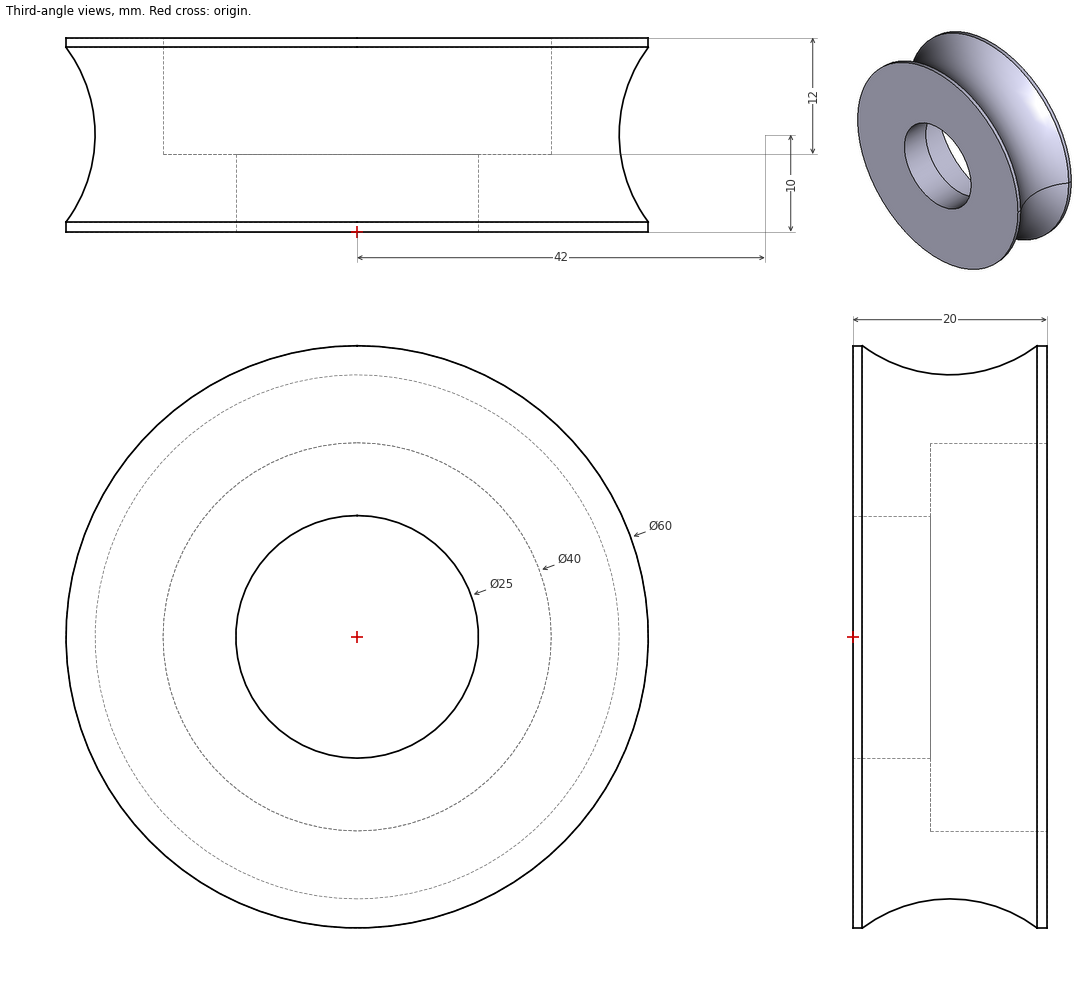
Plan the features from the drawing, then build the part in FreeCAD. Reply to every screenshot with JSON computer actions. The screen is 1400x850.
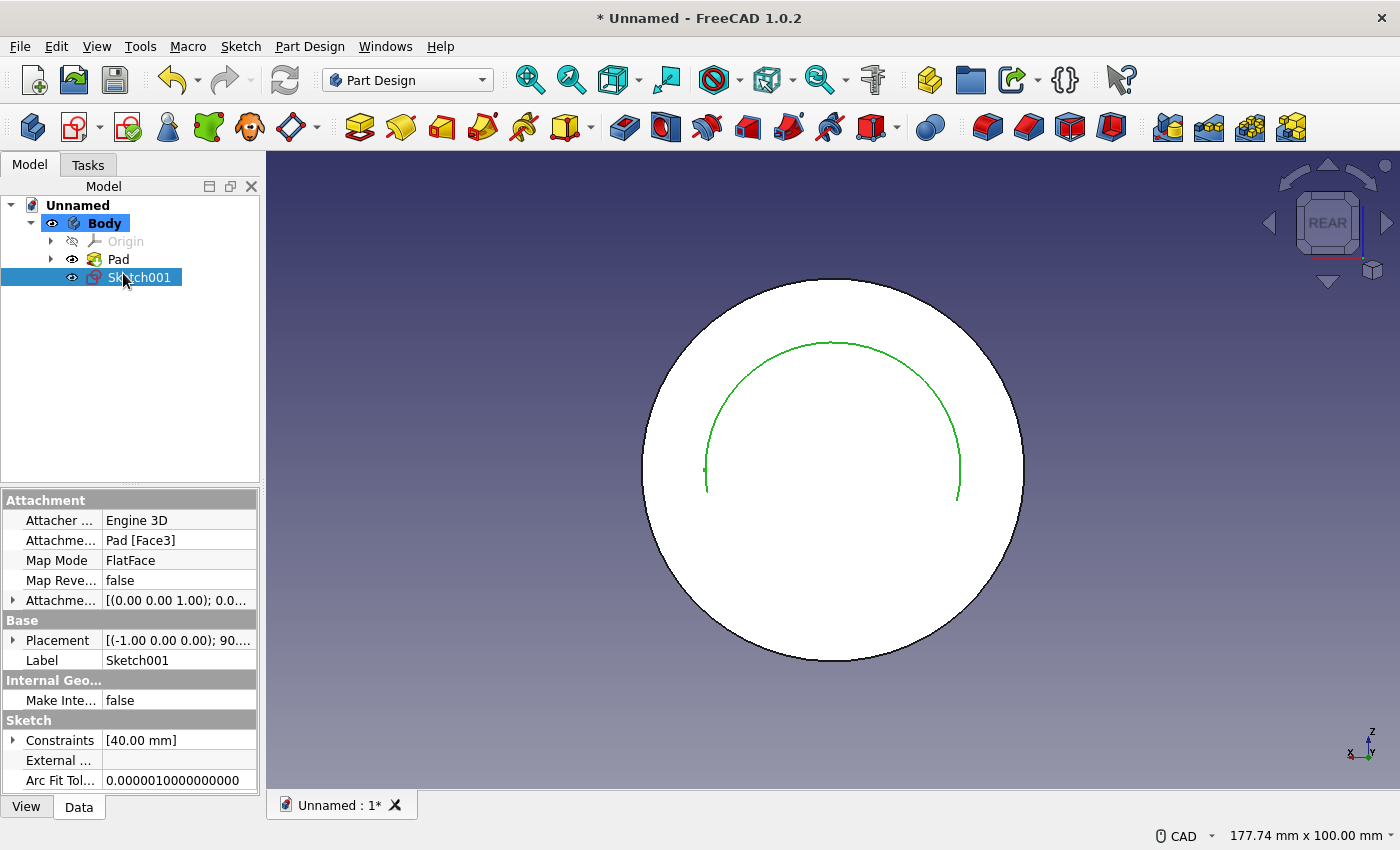
{"action": "left_click", "coordinate": [625, 128]}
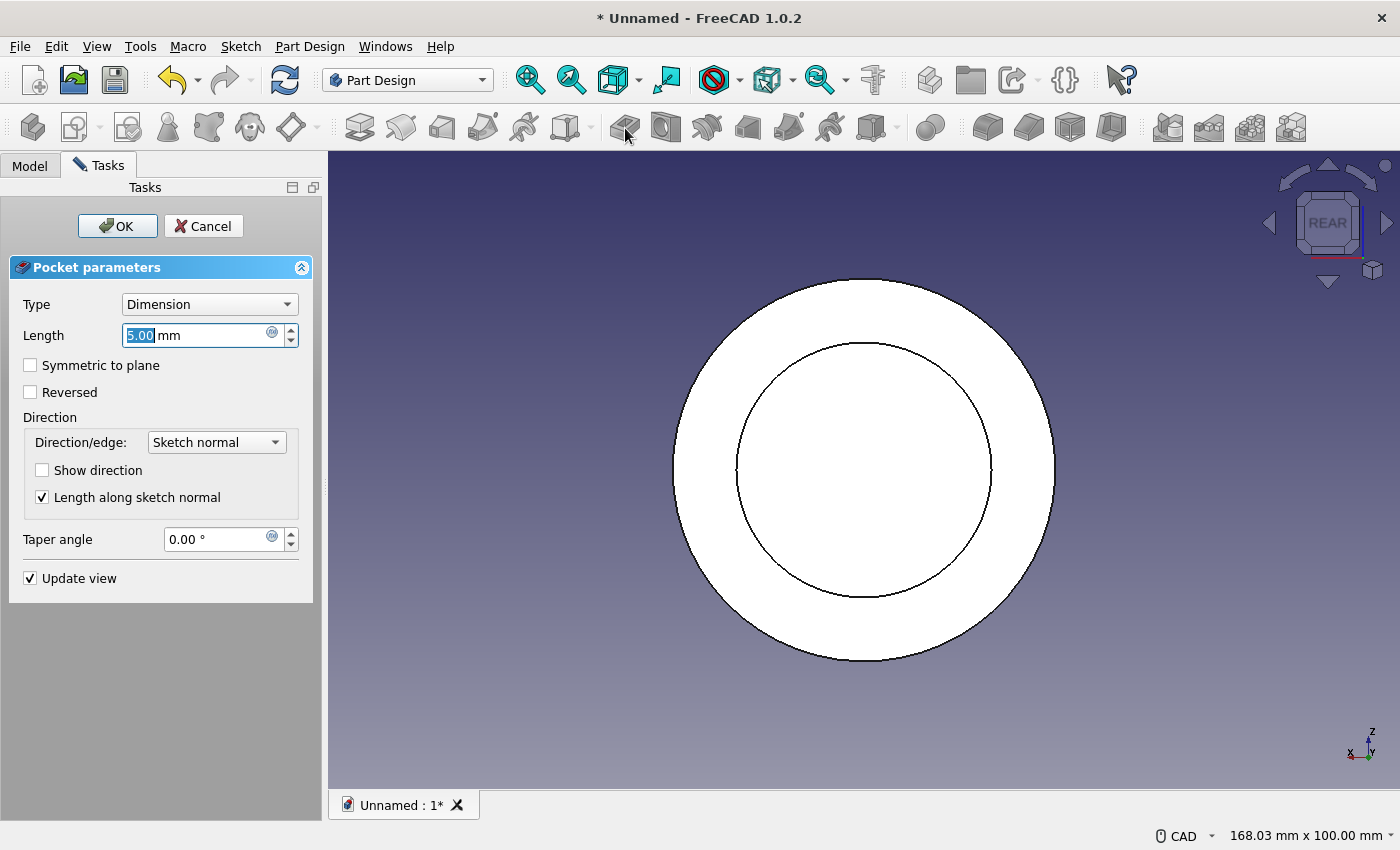
{"action": "type", "text": "12"}
{"action": "key", "text": "Tab"}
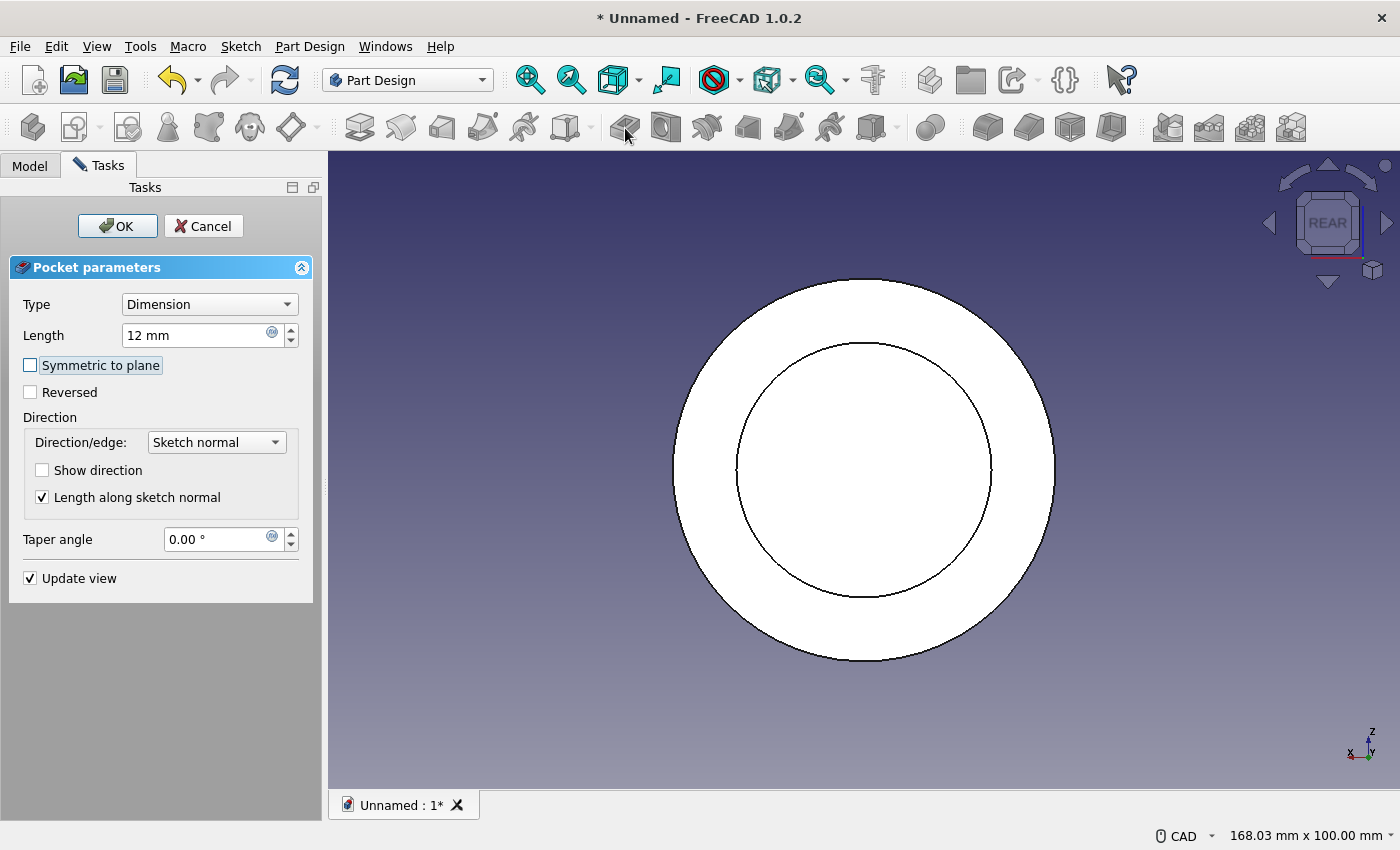
{"action": "left_click", "coordinate": [118, 226]}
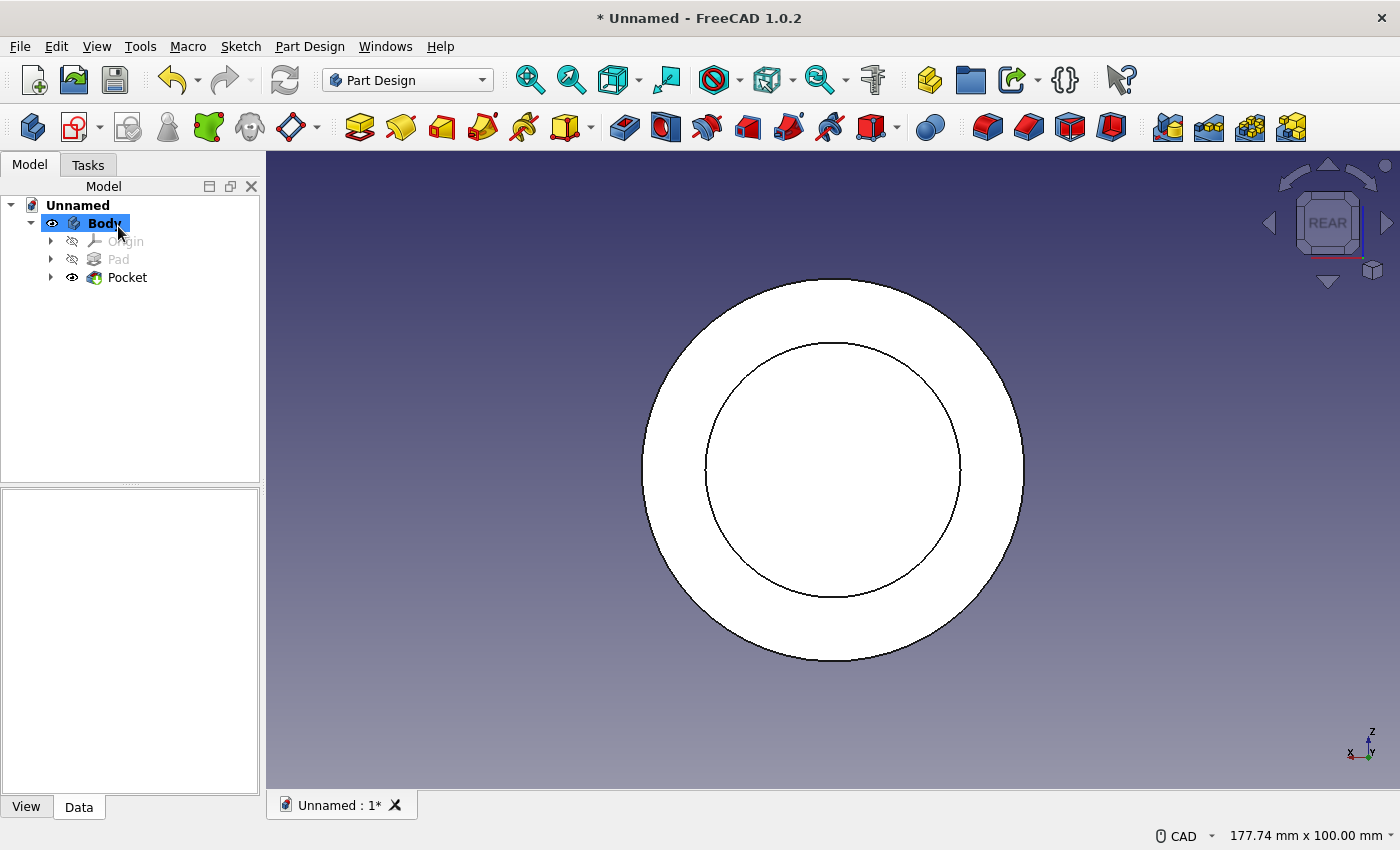
{"action": "left_click", "coordinate": [833, 469]}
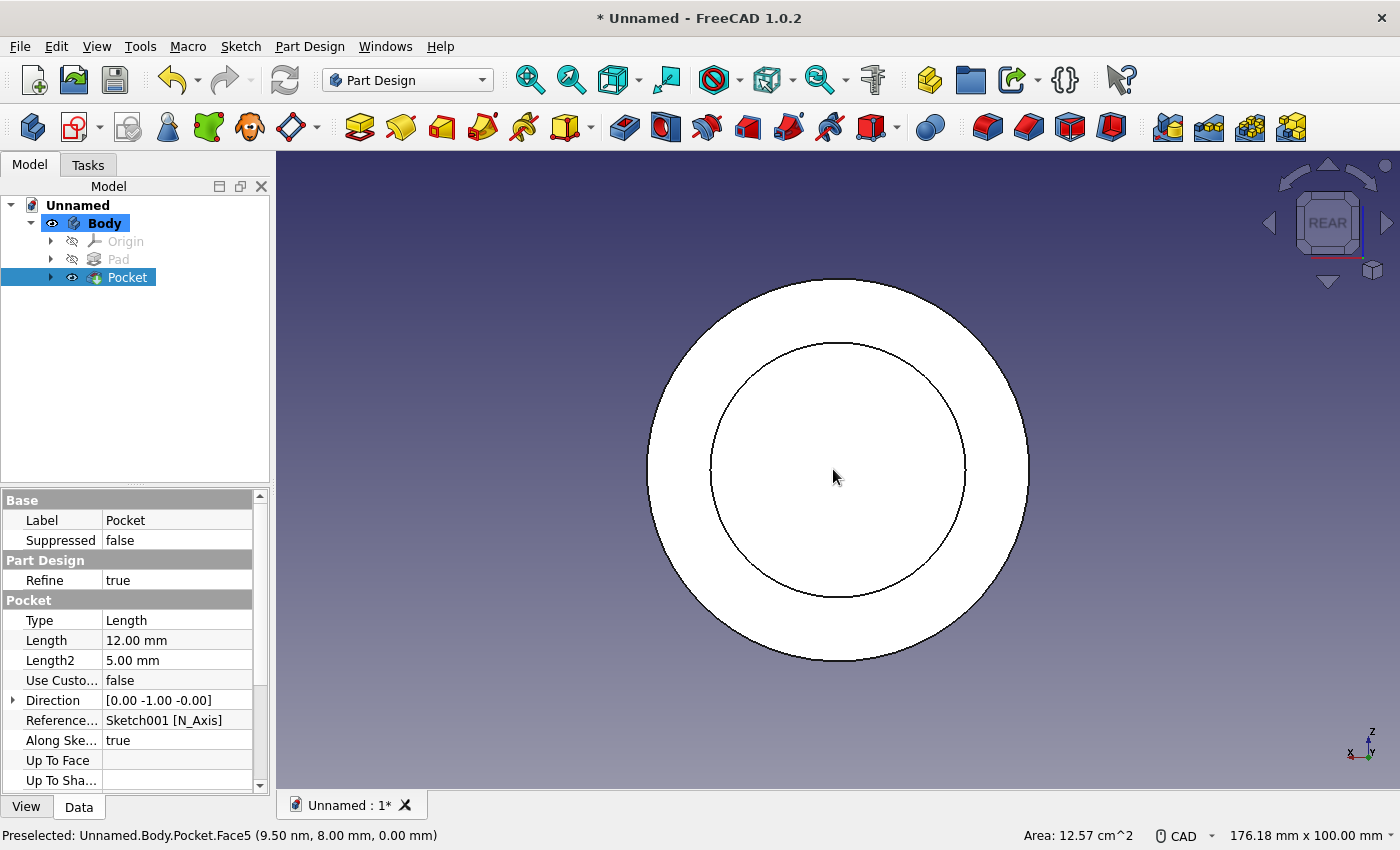
{"action": "left_click", "coordinate": [74, 128]}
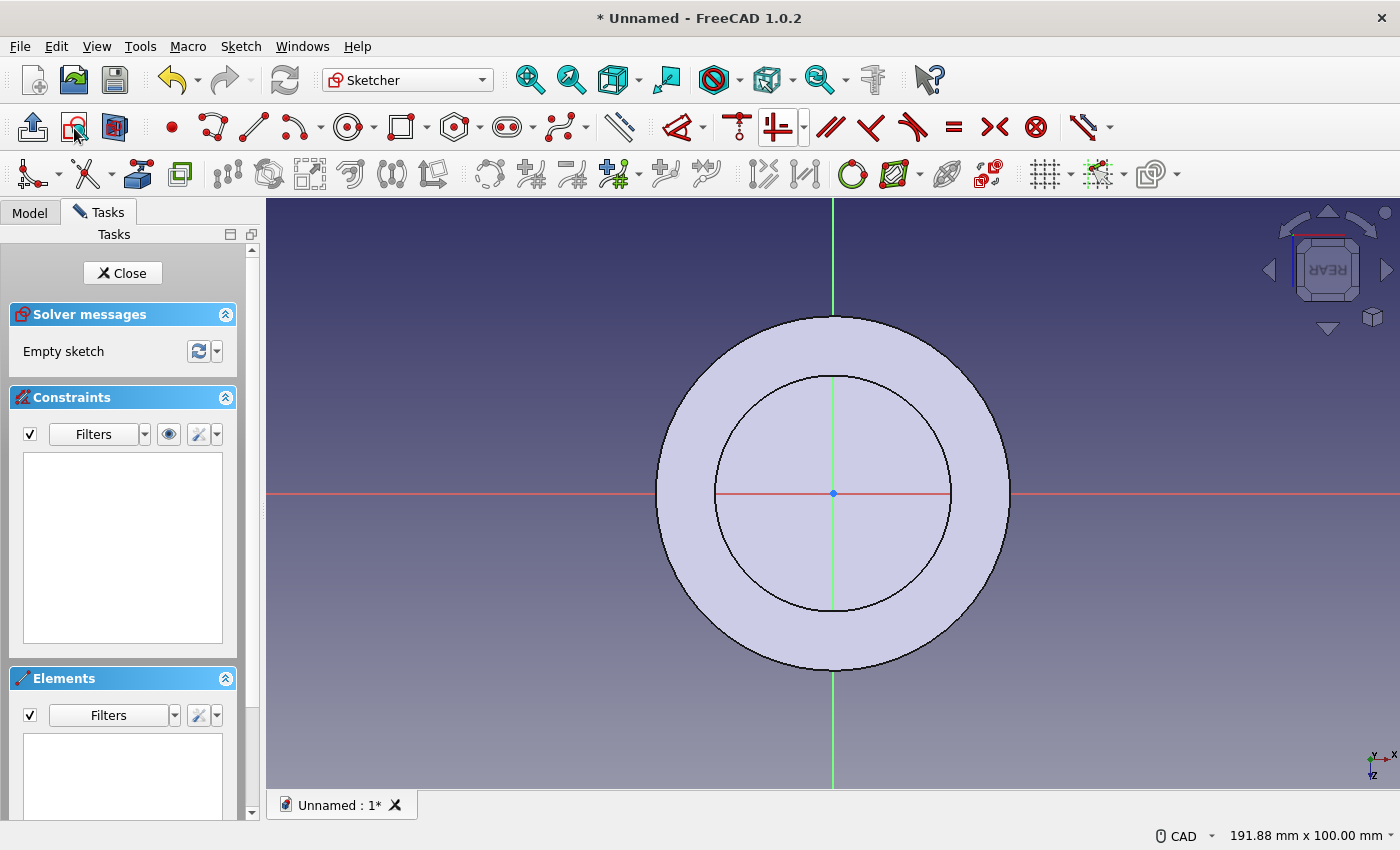
{"action": "scroll", "coordinate": [873, 493], "scroll_direction": "up", "scroll_amount": 5}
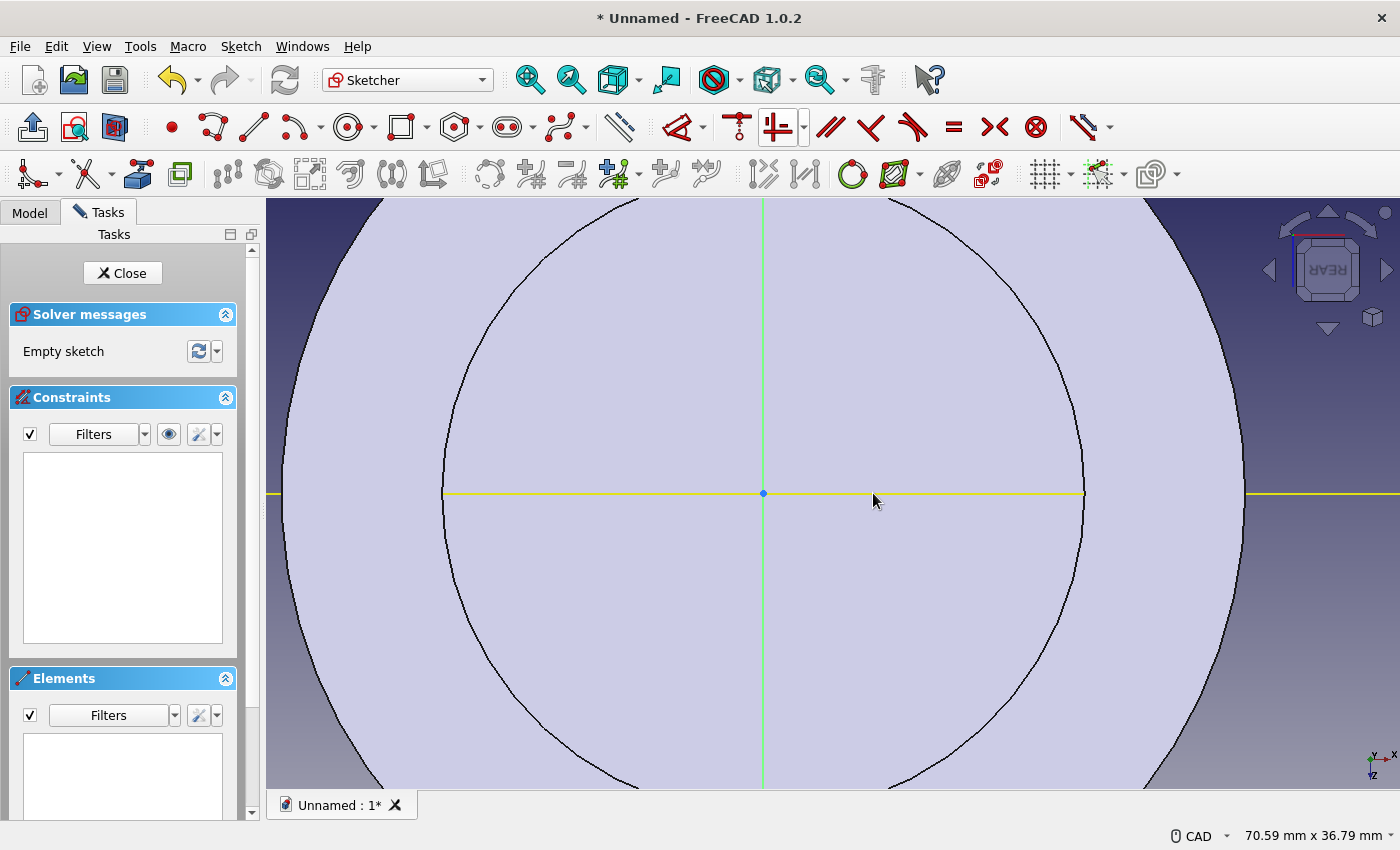
{"action": "left_click", "coordinate": [348, 128]}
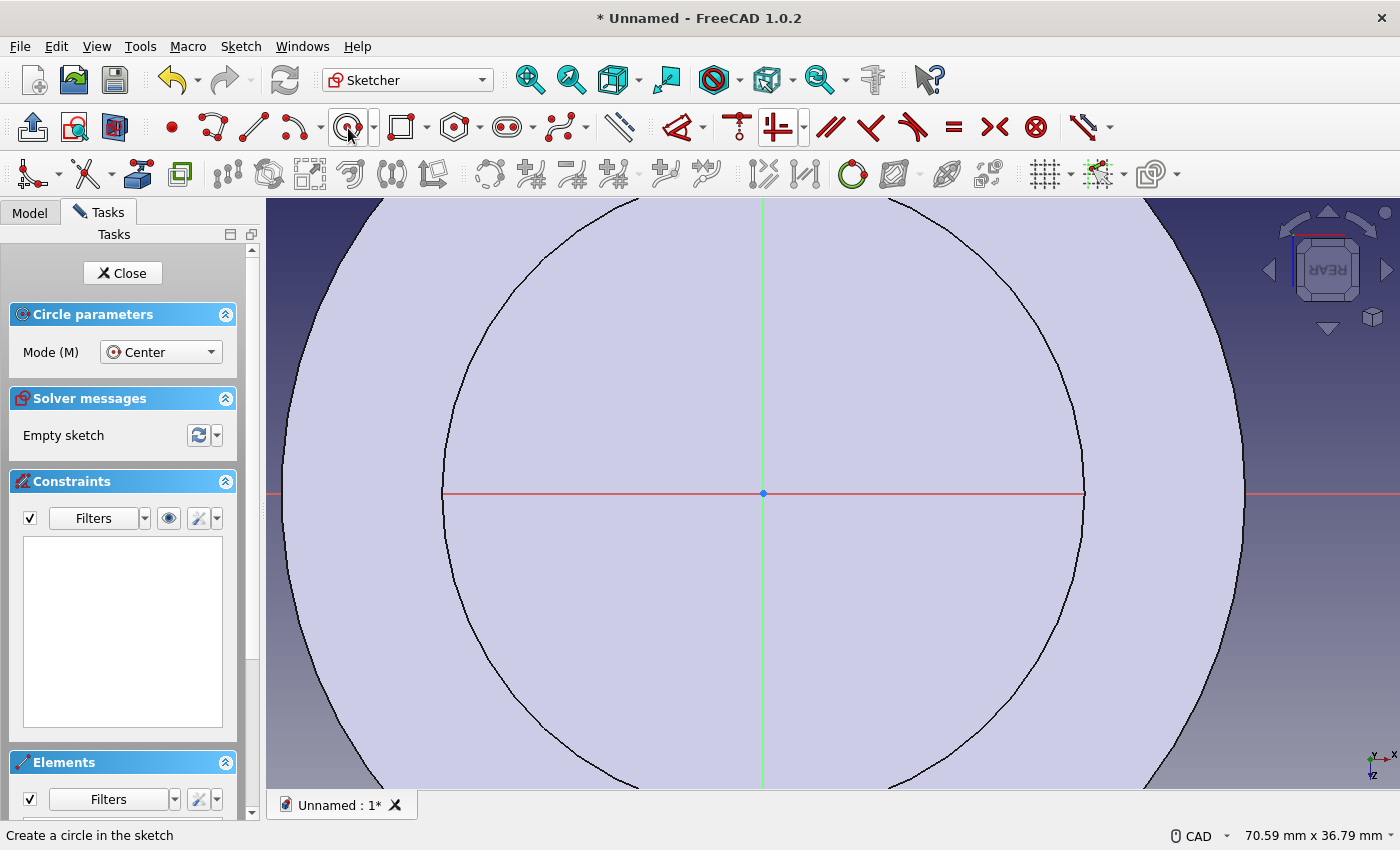
{"action": "left_click", "coordinate": [763, 493]}
{"action": "left_click", "coordinate": [905, 352]}
{"action": "key", "text": "Escape"}